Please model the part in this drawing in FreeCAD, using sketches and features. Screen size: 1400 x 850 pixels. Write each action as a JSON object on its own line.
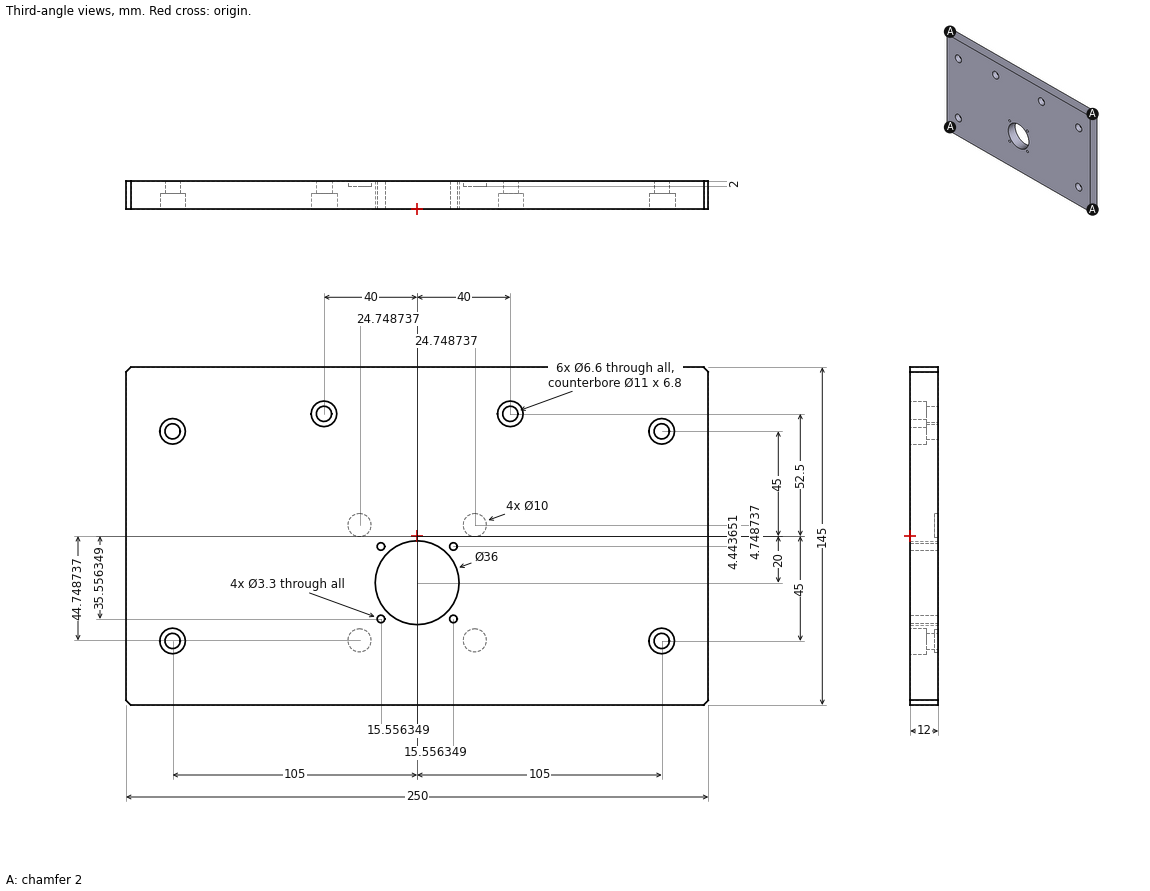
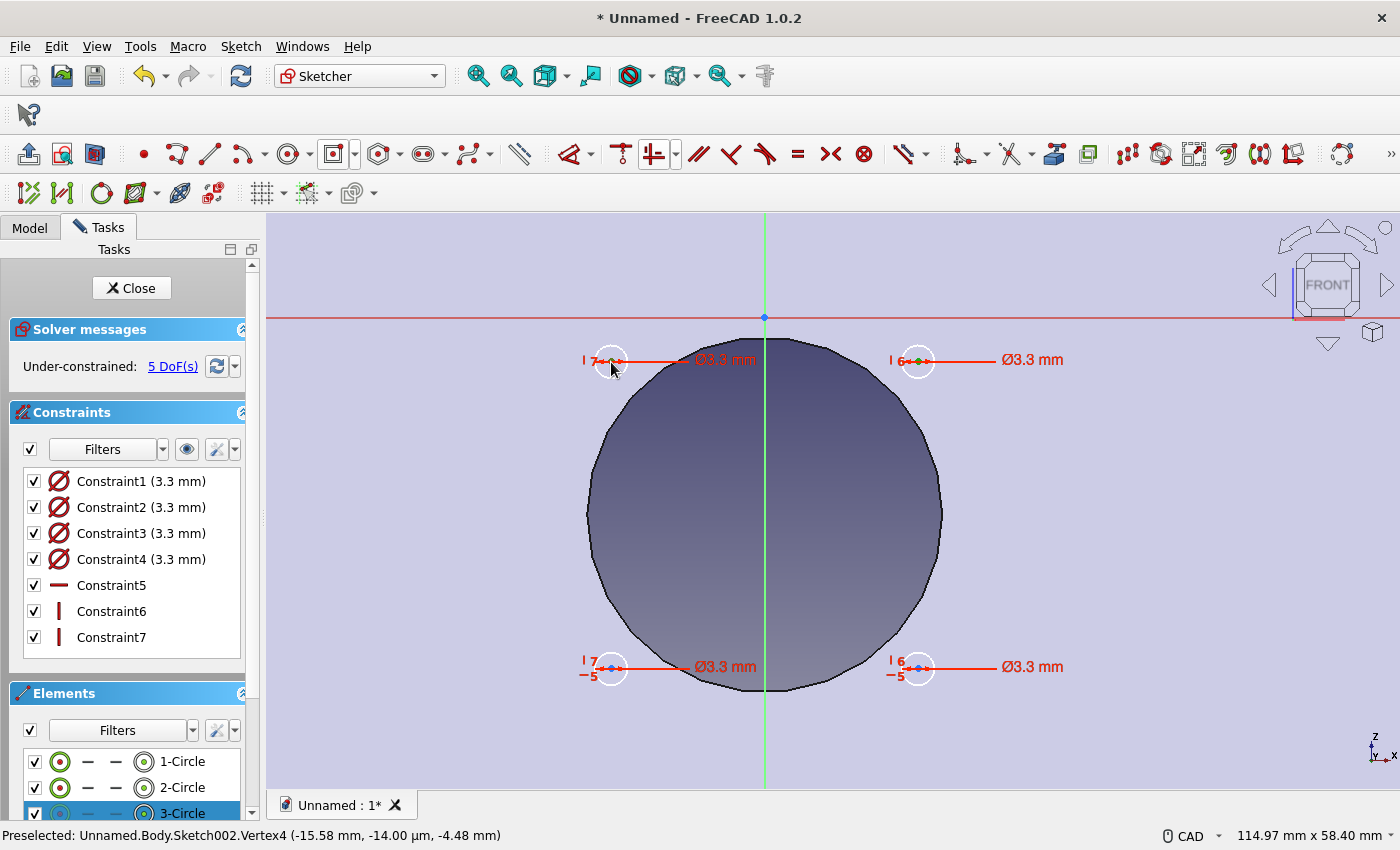
{"action": "key", "text": "h"}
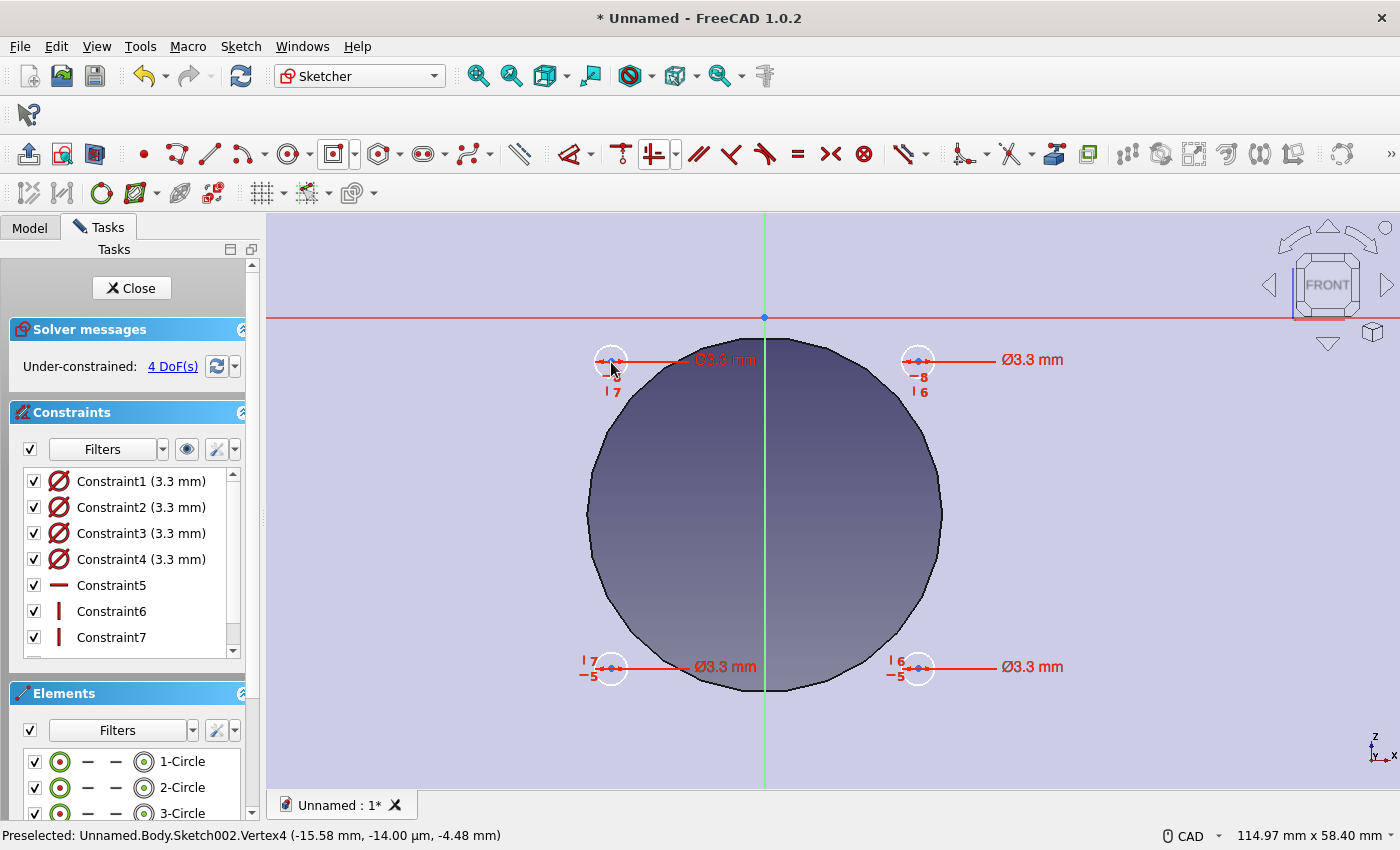
{"action": "left_click", "coordinate": [568, 154]}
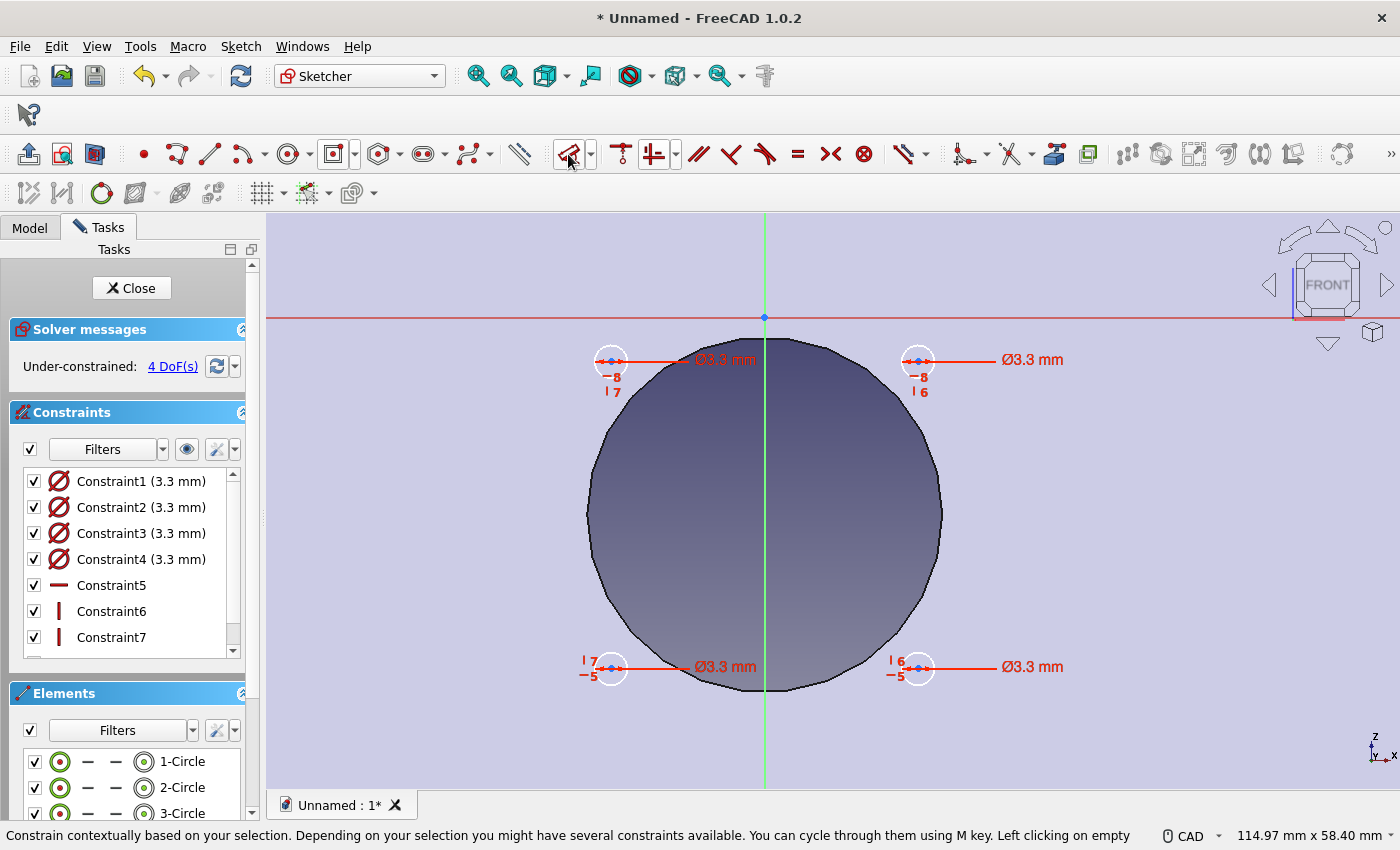
{"action": "left_click", "coordinate": [918, 362]}
{"action": "left_click", "coordinate": [952, 340]}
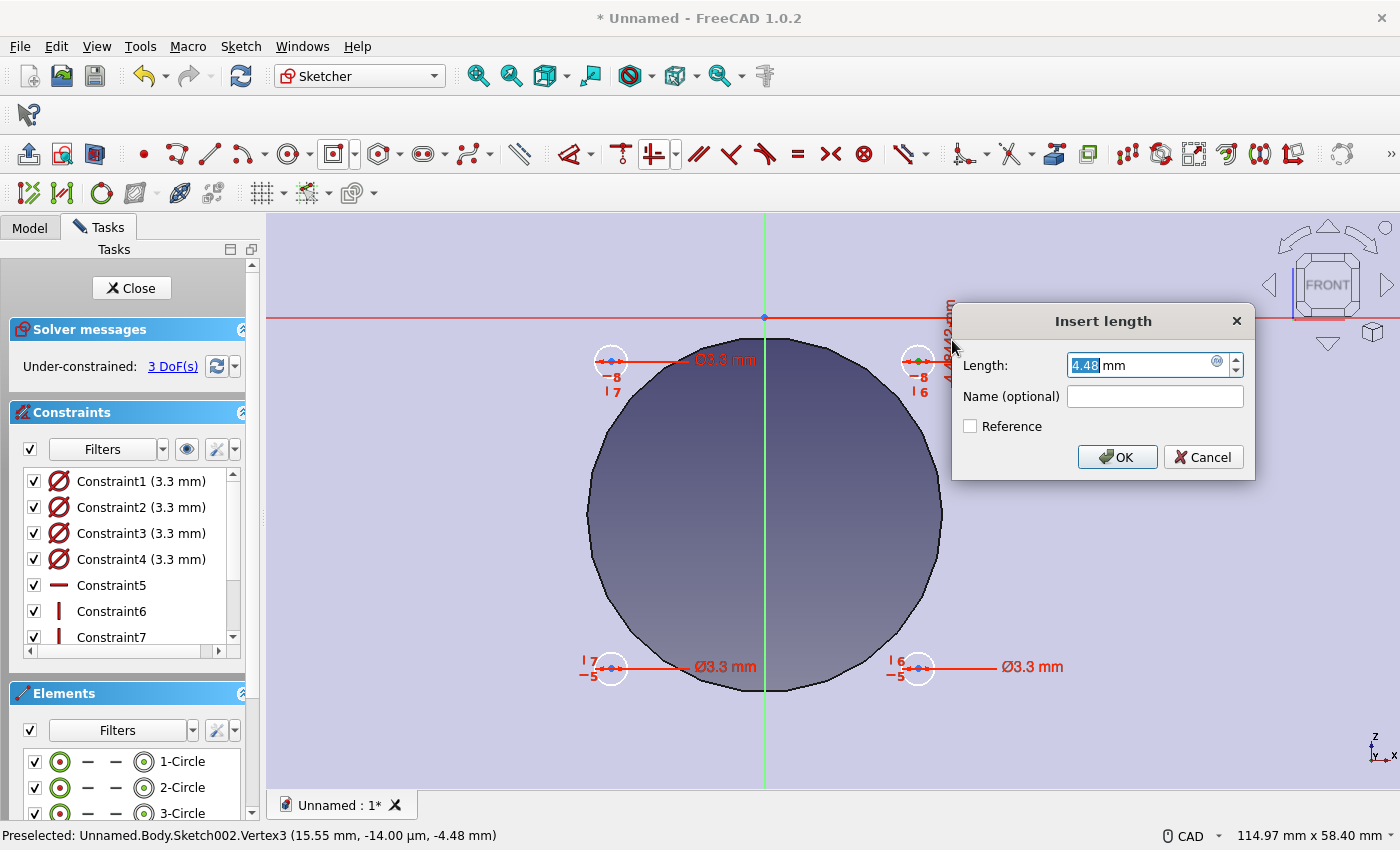
{"action": "type", "text": "4.443651"}
{"action": "key", "text": "Return"}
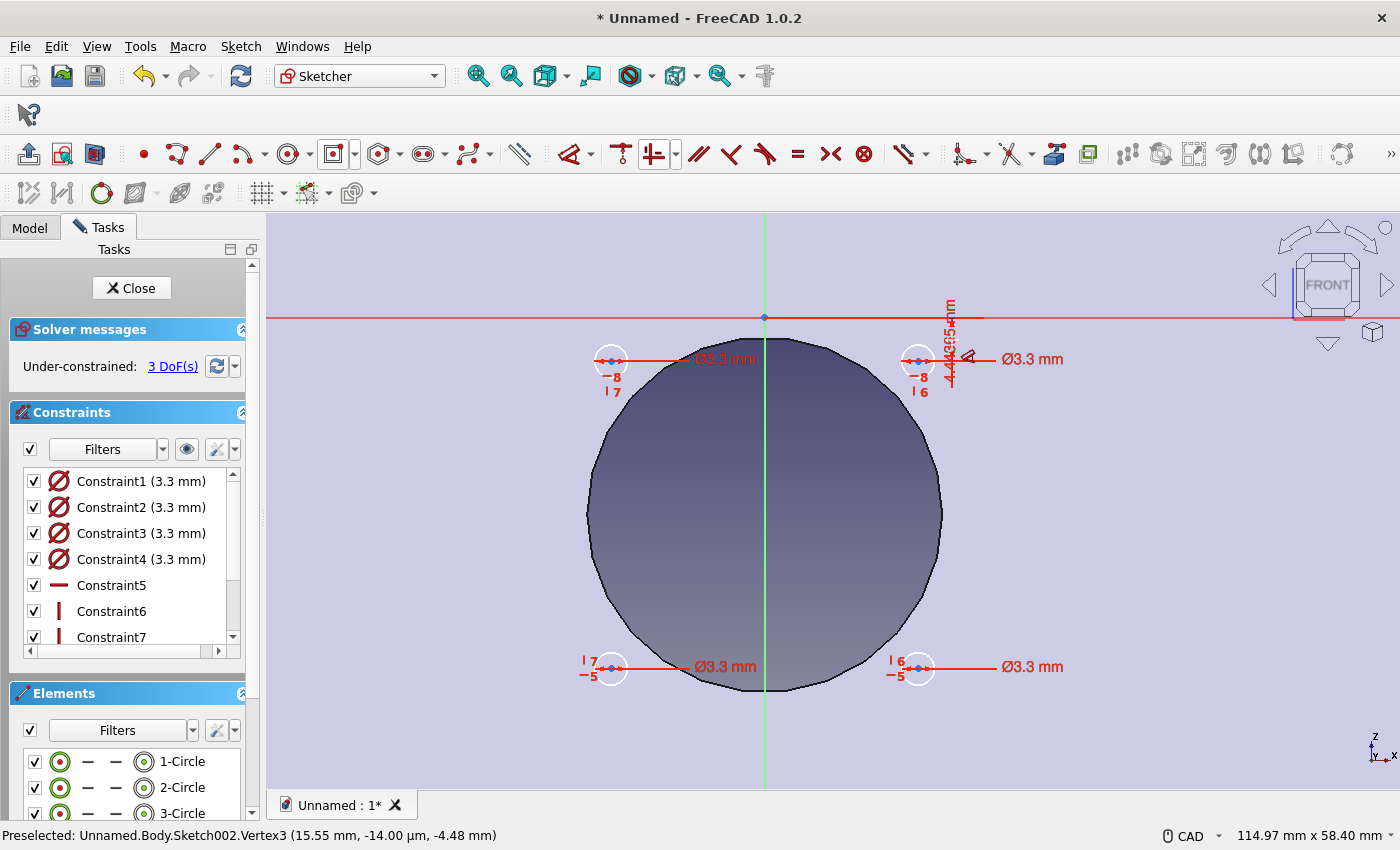
{"action": "left_click", "coordinate": [611, 669]}
{"action": "left_click", "coordinate": [688, 284]}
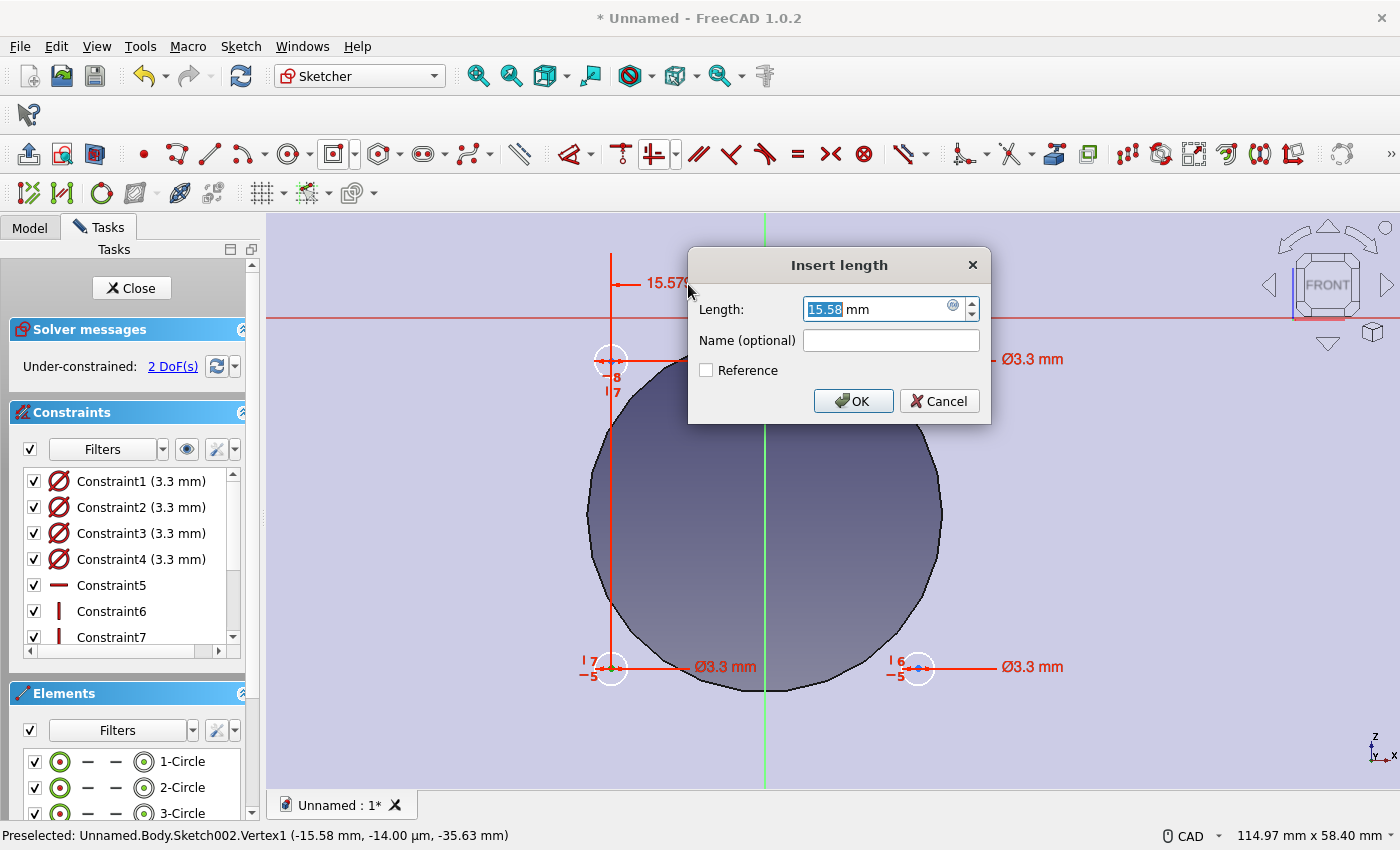
{"action": "type", "text": "15.556349"}
{"action": "key", "text": "Return"}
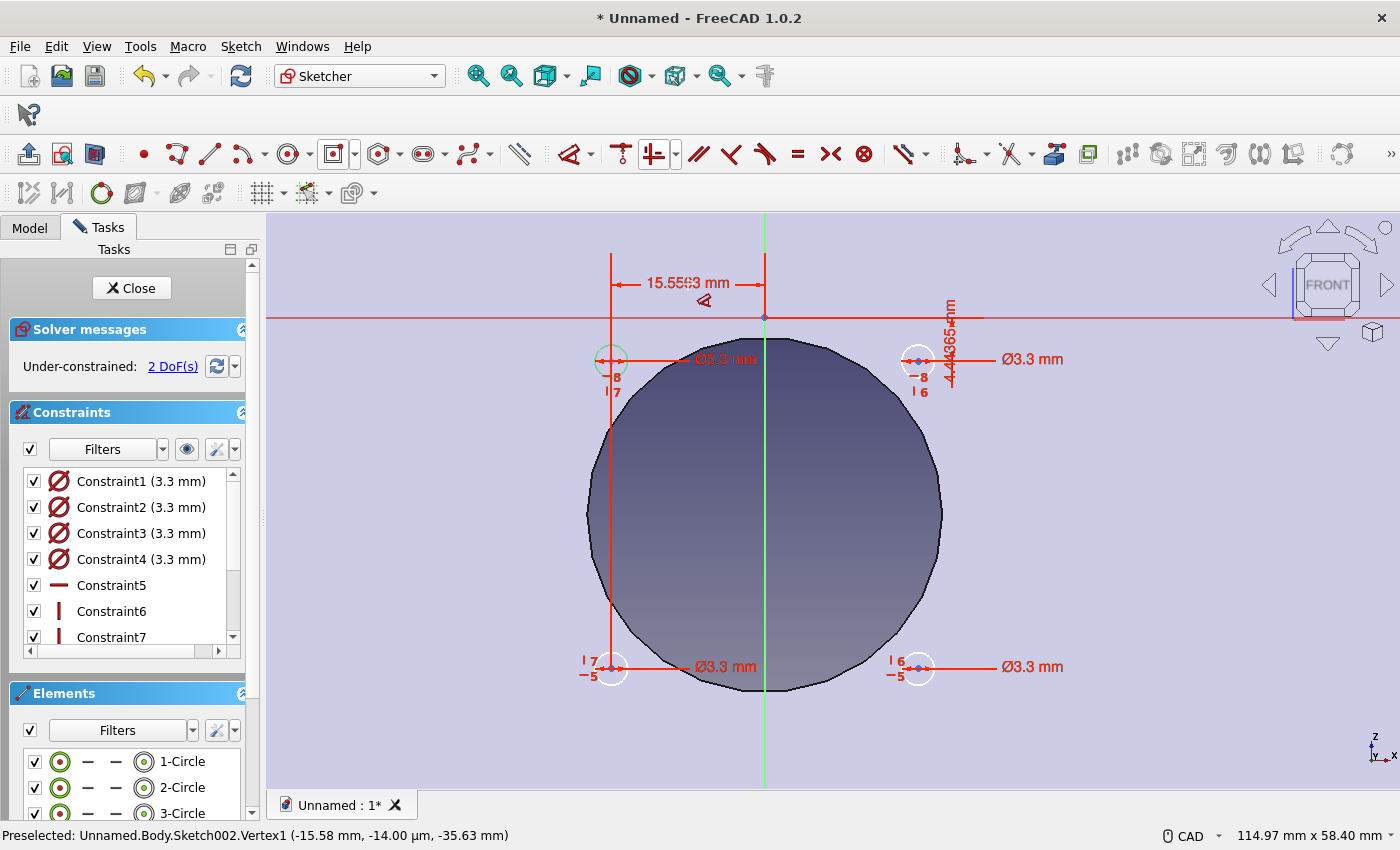
{"action": "left_click", "coordinate": [611, 669]}
{"action": "left_click", "coordinate": [577, 493]}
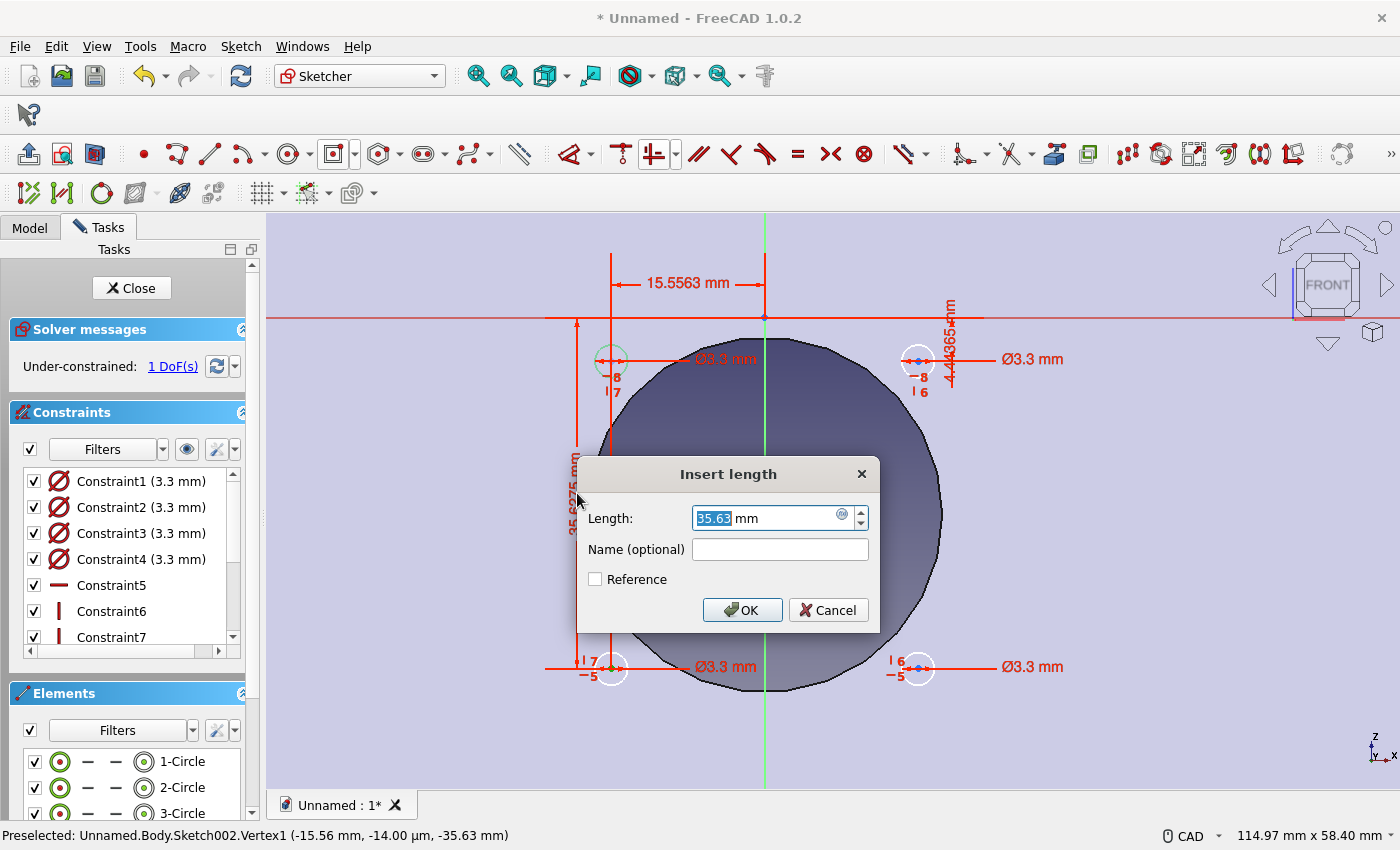
{"action": "type", "text": "35.556349"}
{"action": "key", "text": "Return"}